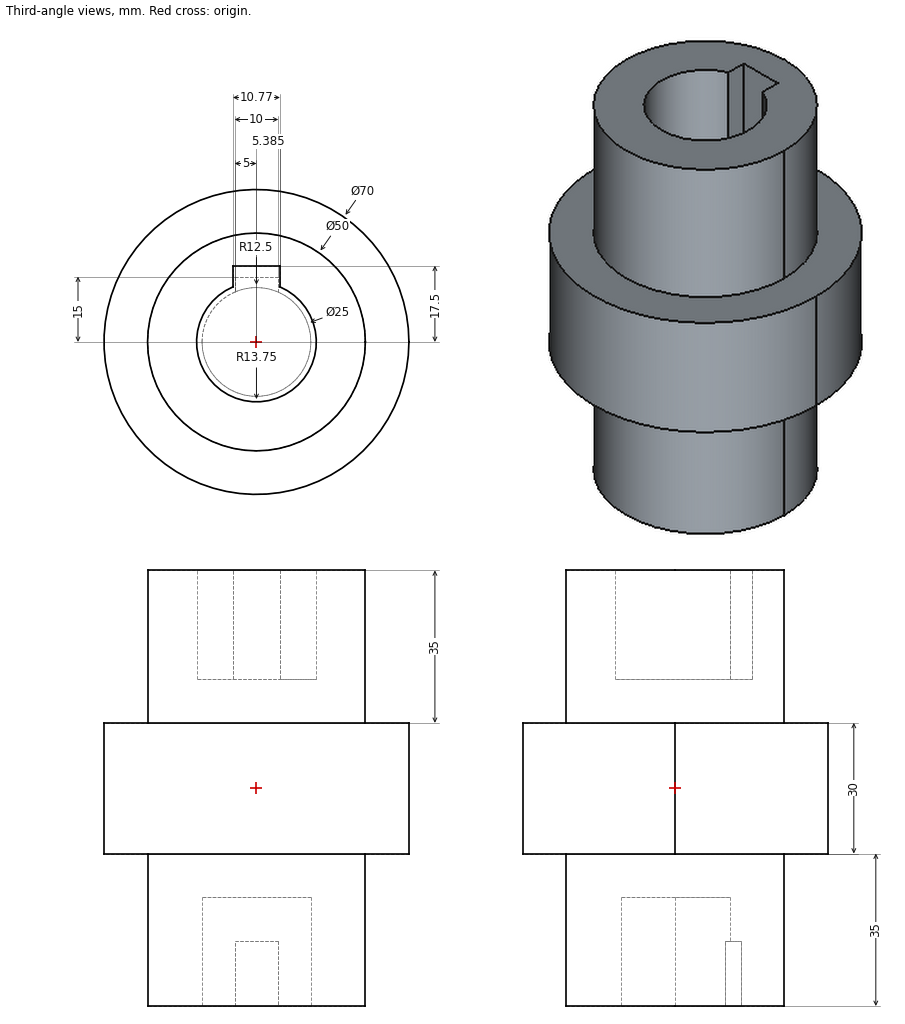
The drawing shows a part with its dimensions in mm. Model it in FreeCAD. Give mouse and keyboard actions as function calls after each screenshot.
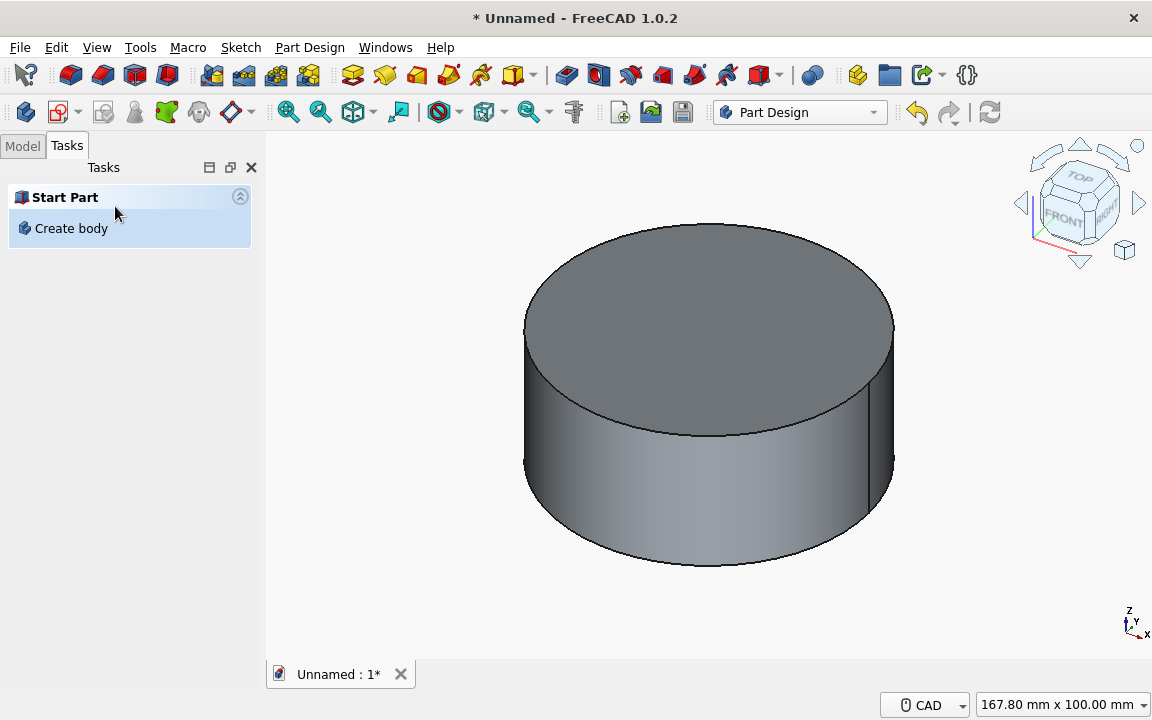
click(709, 329)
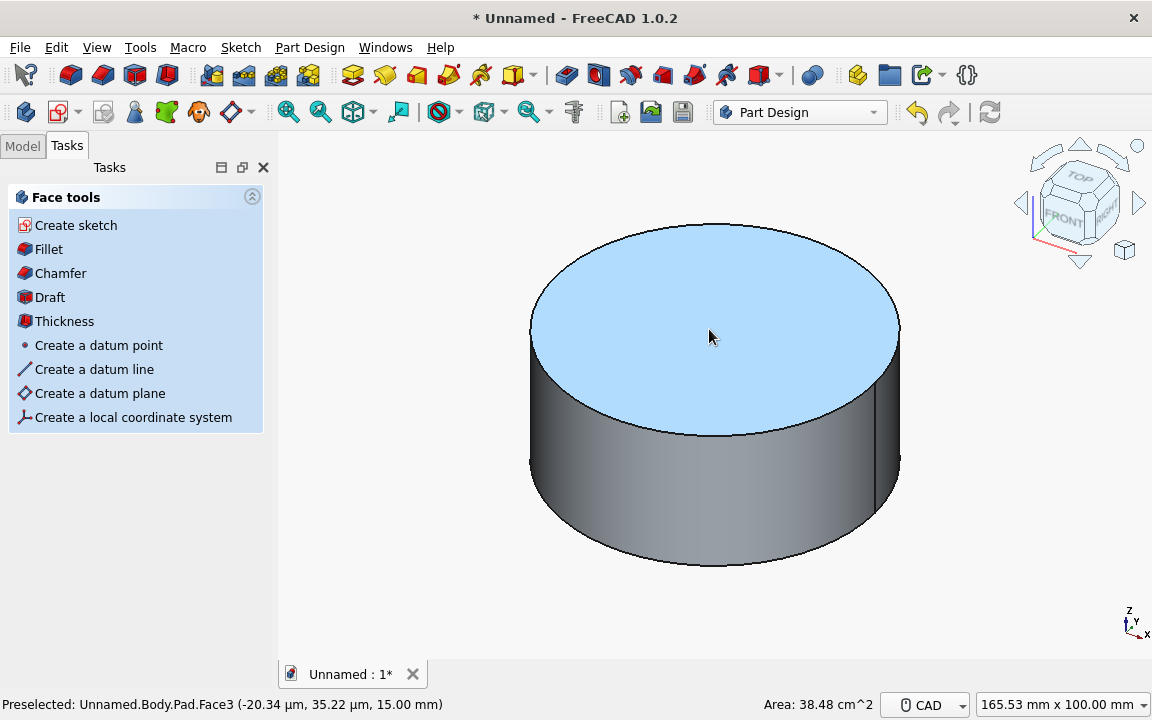
click(58, 112)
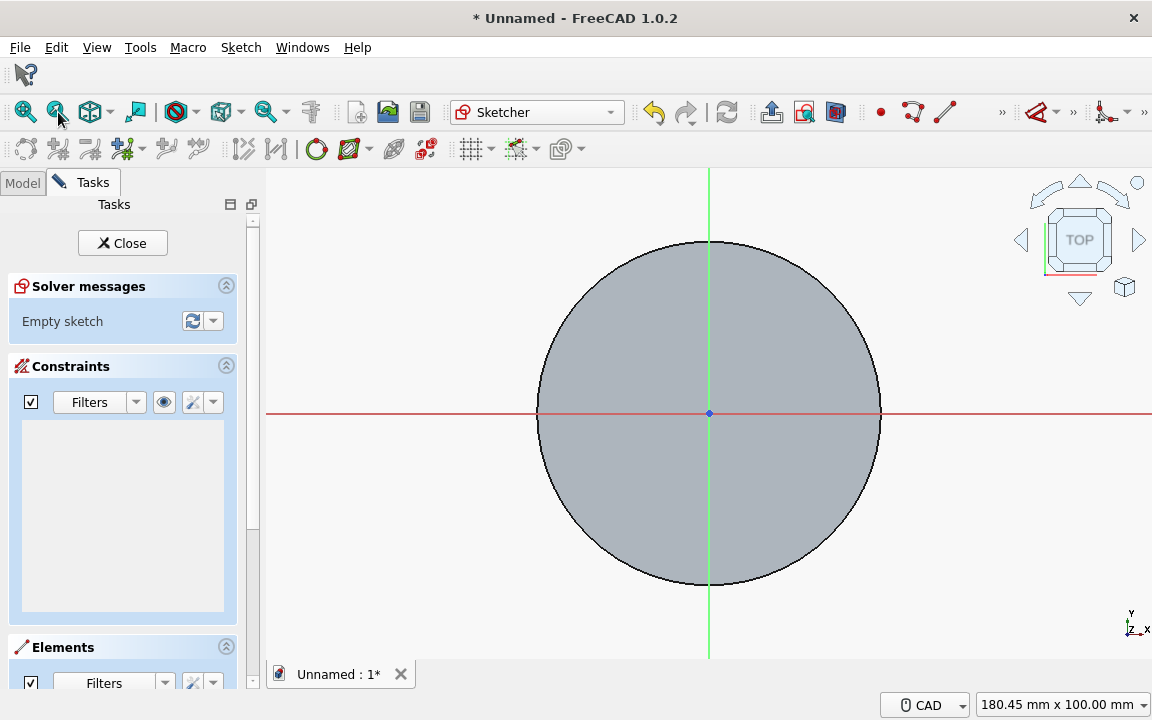
key(g)
key(c)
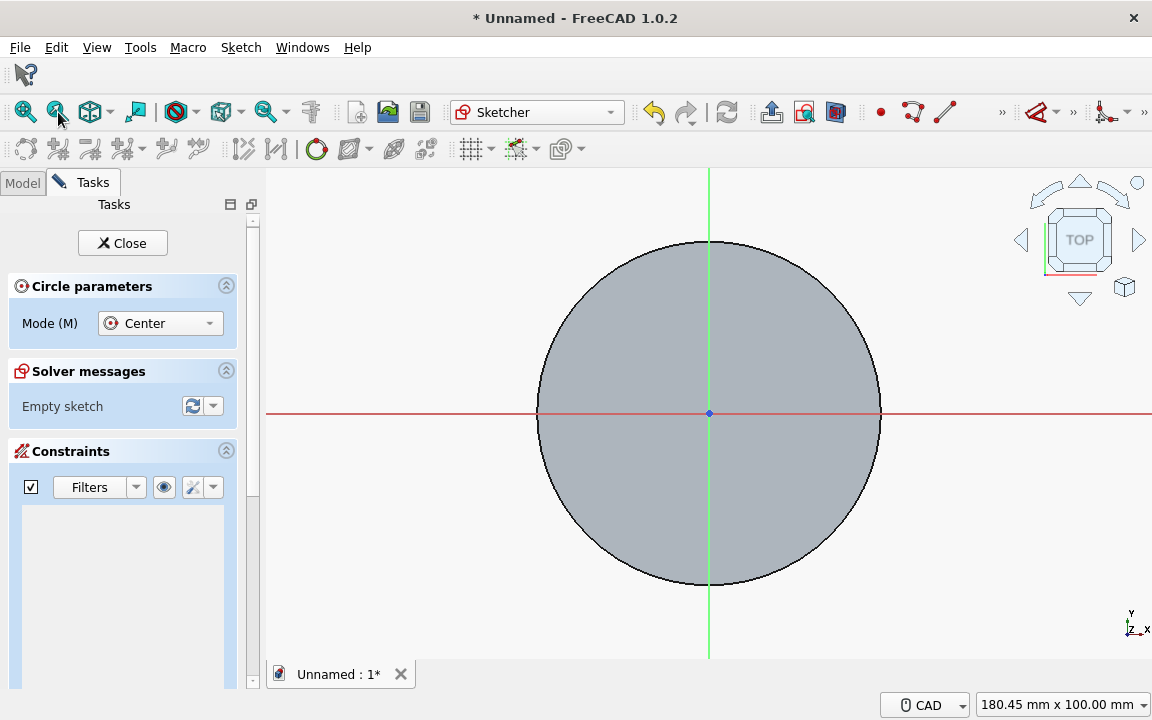
click(709, 414)
move(796, 327)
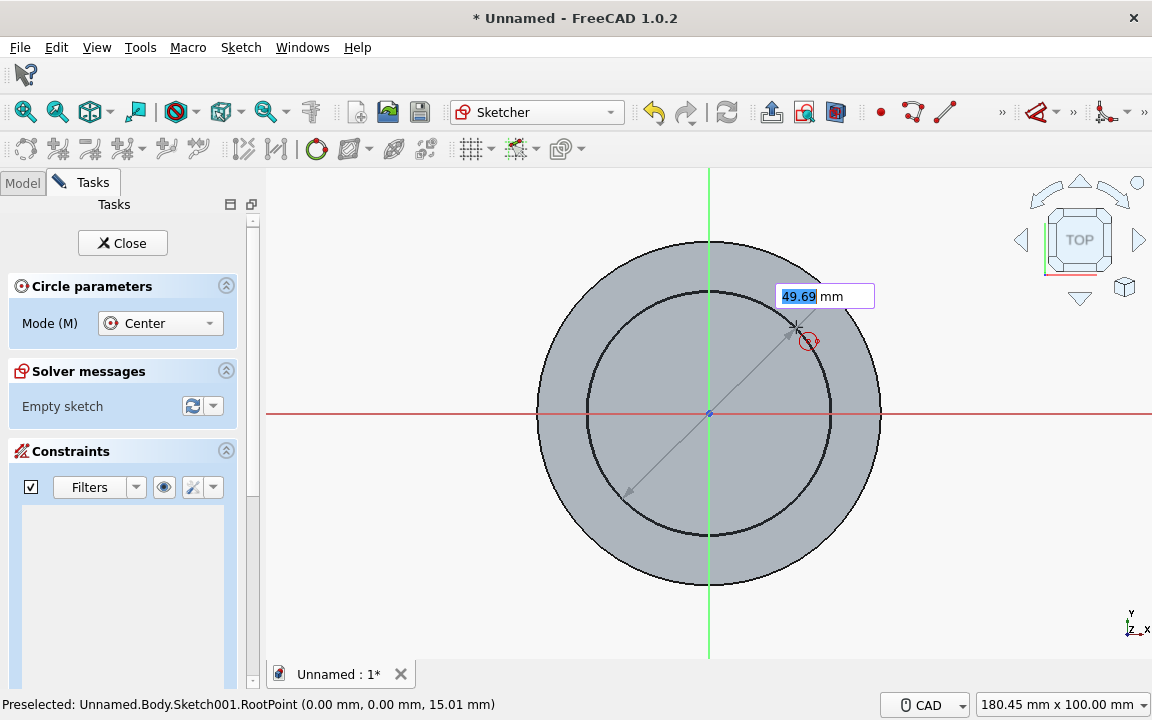
text(50)
key(Return)
key(Escape)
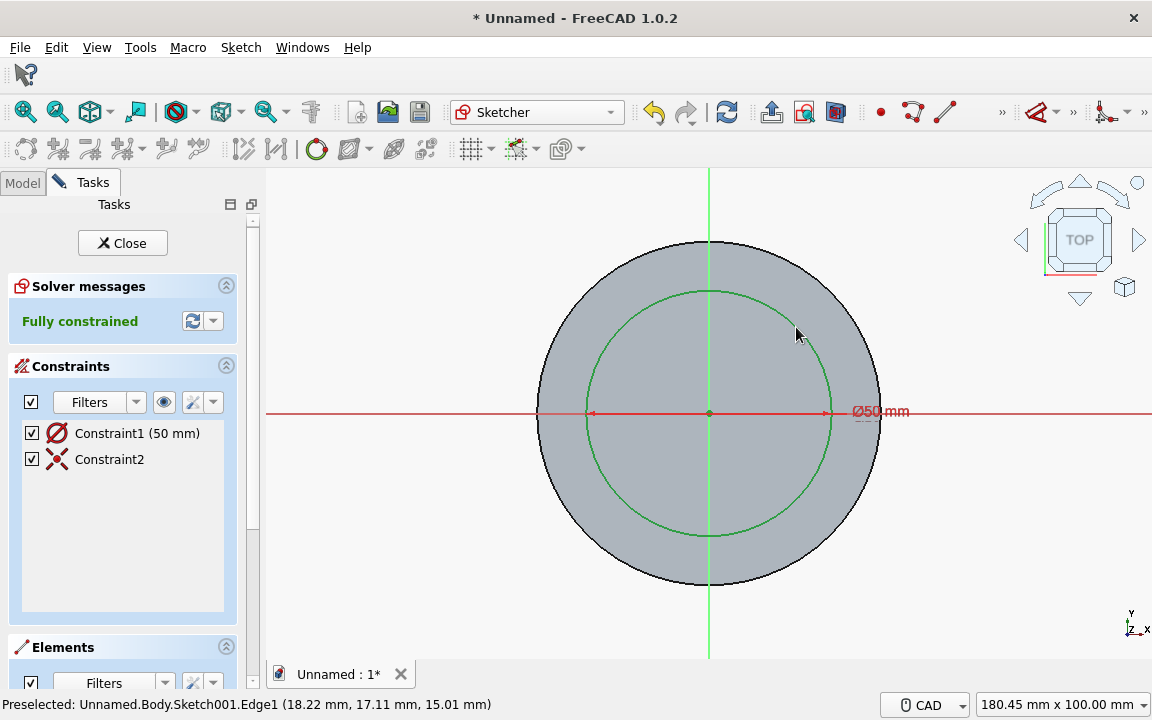
click(123, 243)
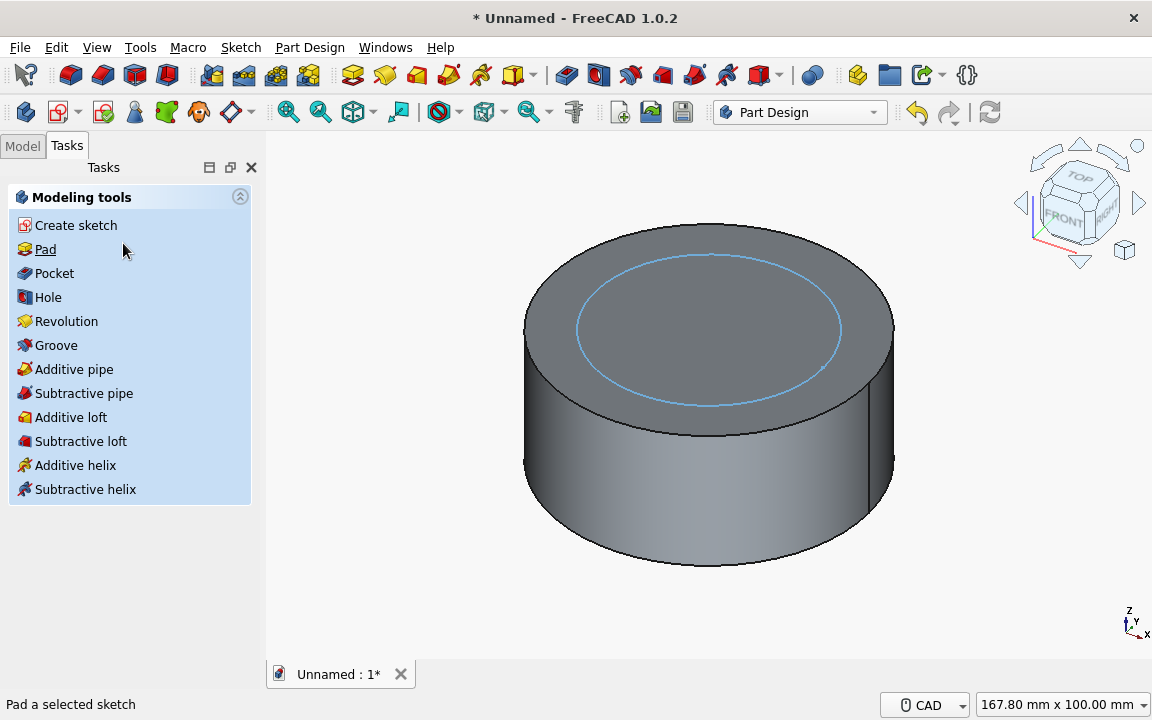
click(354, 76)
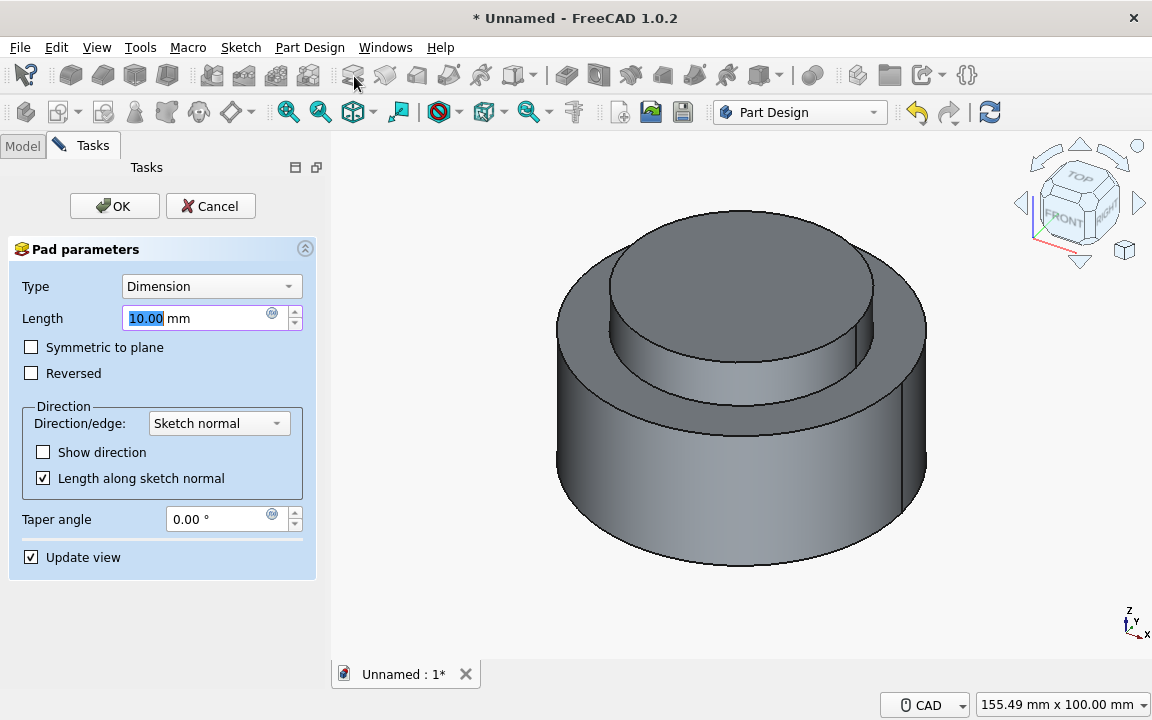
text(35)
key(Tab)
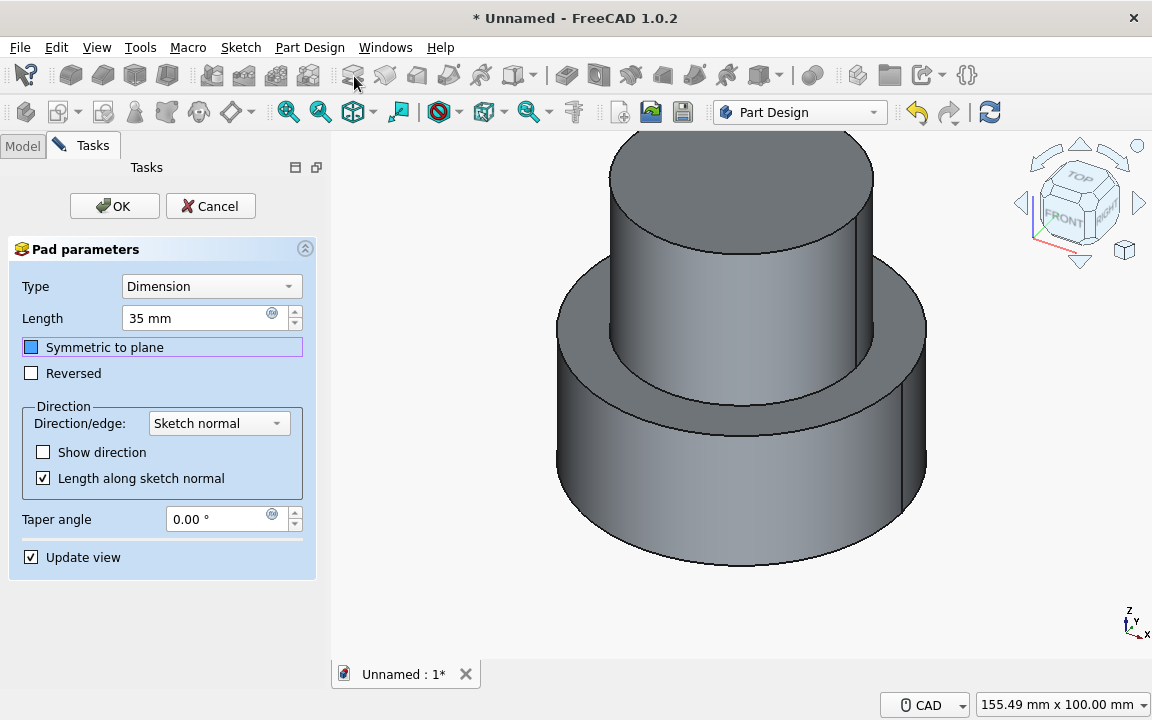
click(115, 206)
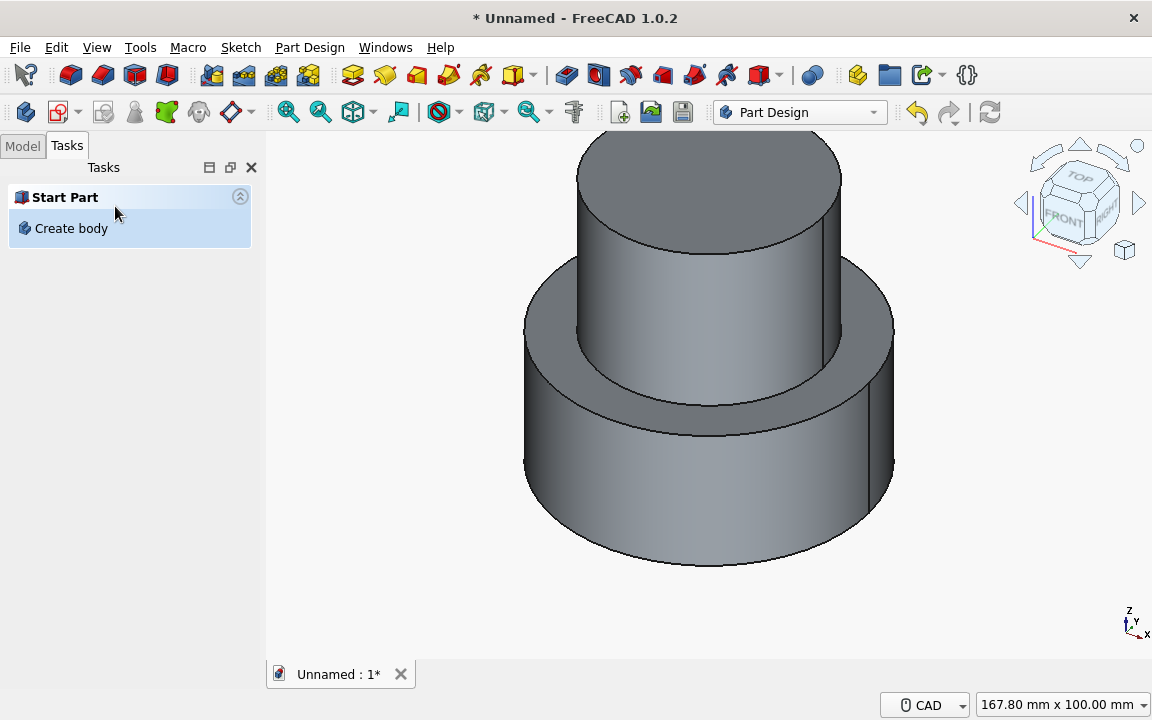
key(v)
key(f)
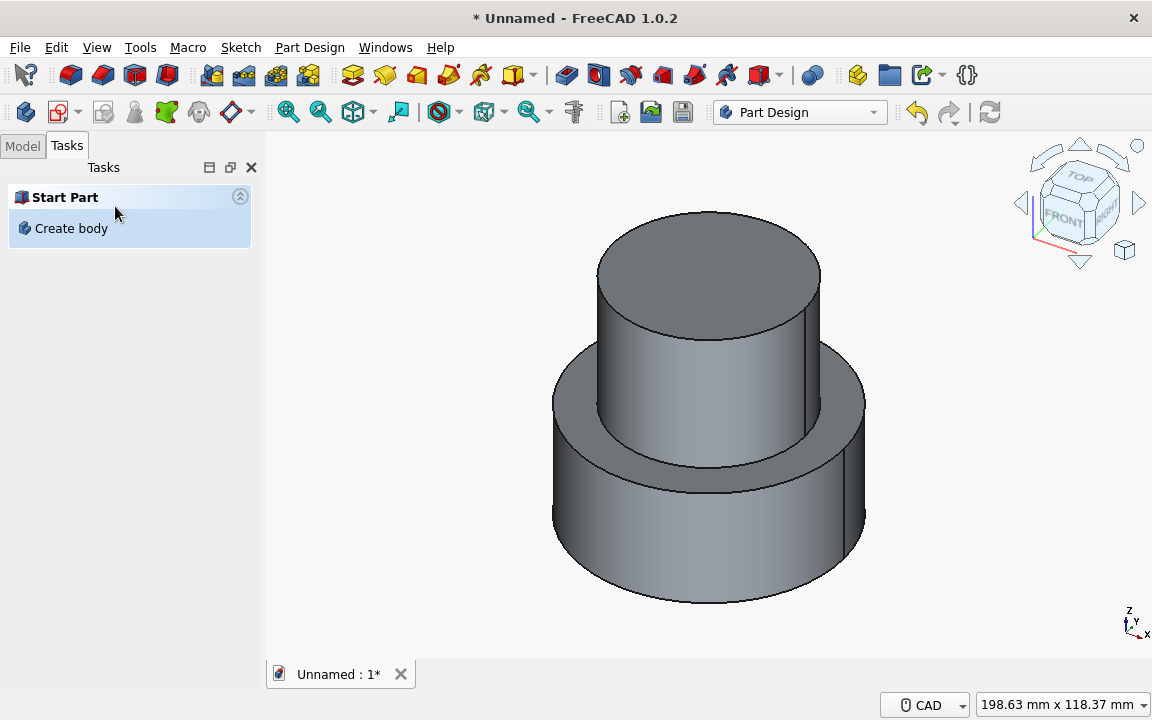
click(23, 145)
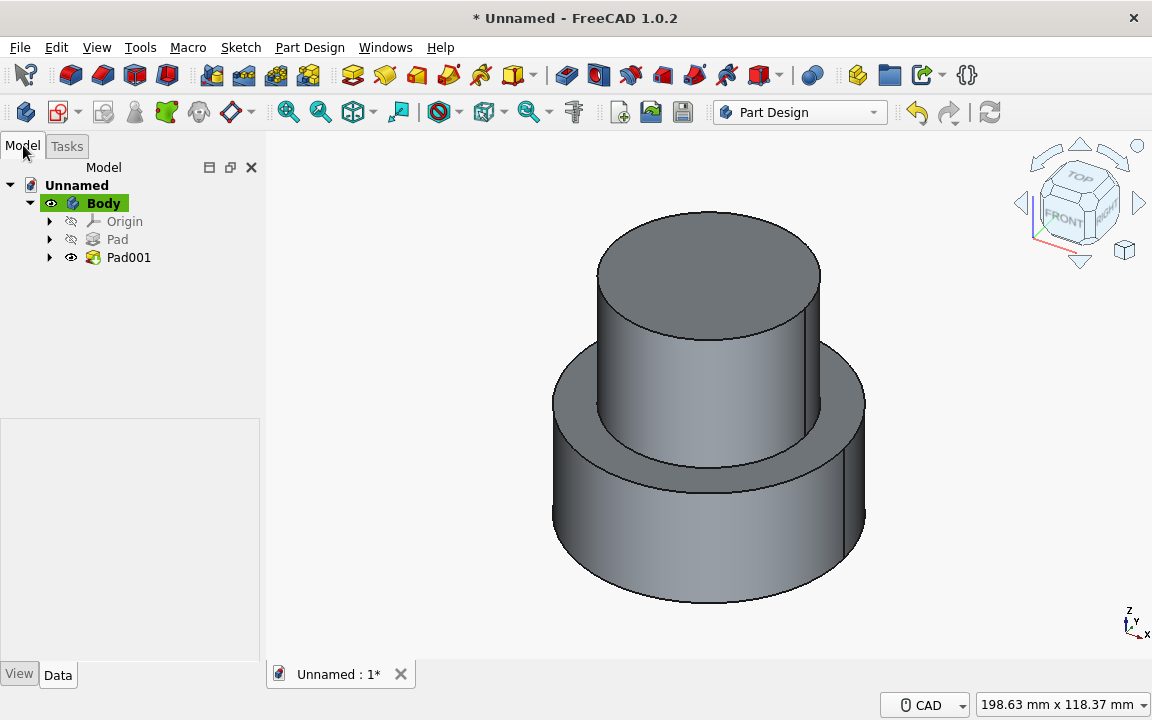
click(50, 221)